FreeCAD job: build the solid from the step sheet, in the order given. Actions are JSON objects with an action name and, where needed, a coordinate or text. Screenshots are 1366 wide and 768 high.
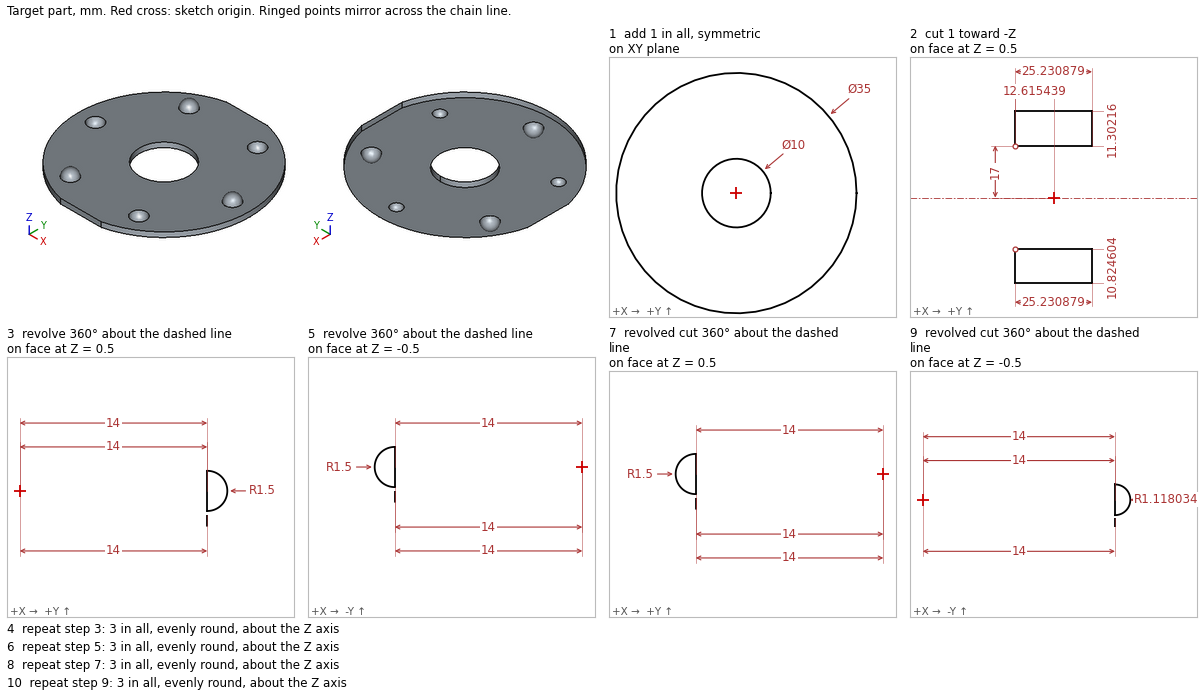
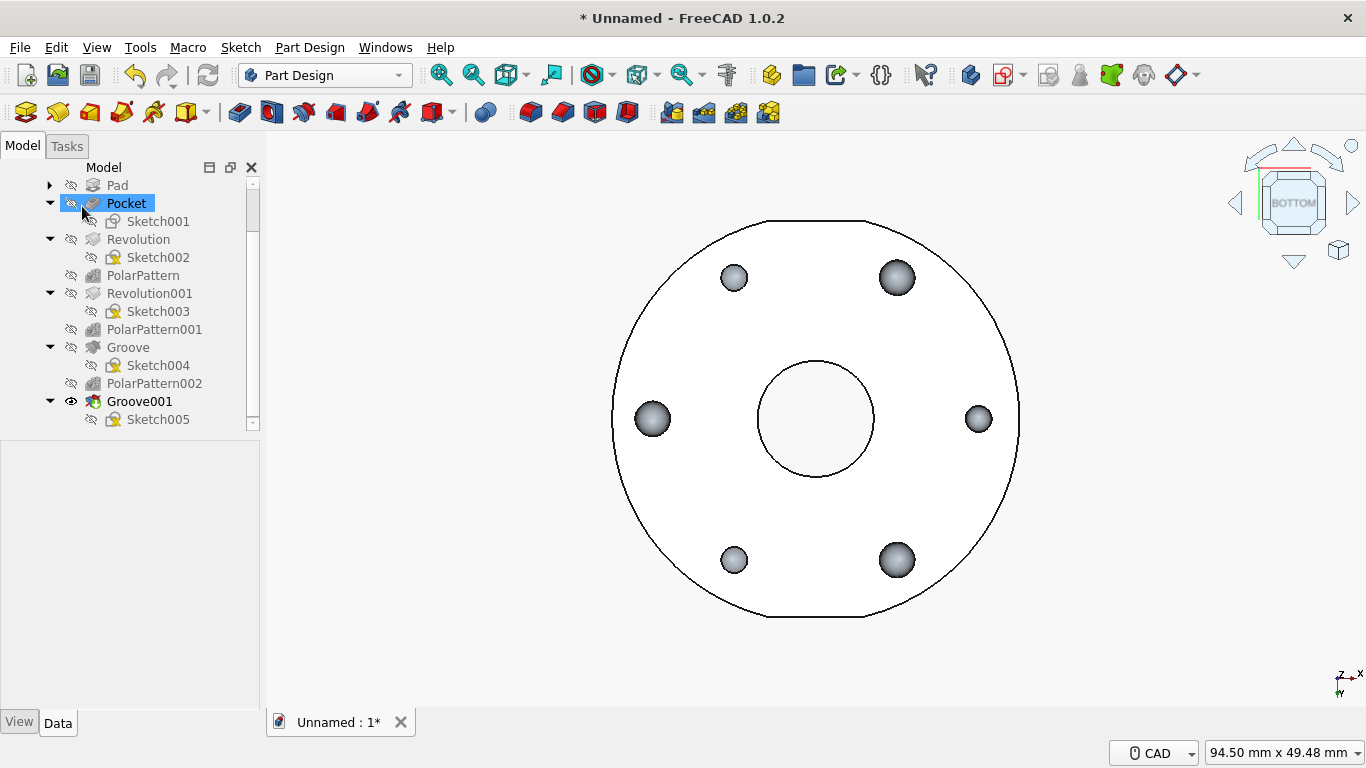
{"action": "left_click", "coordinate": [116, 401]}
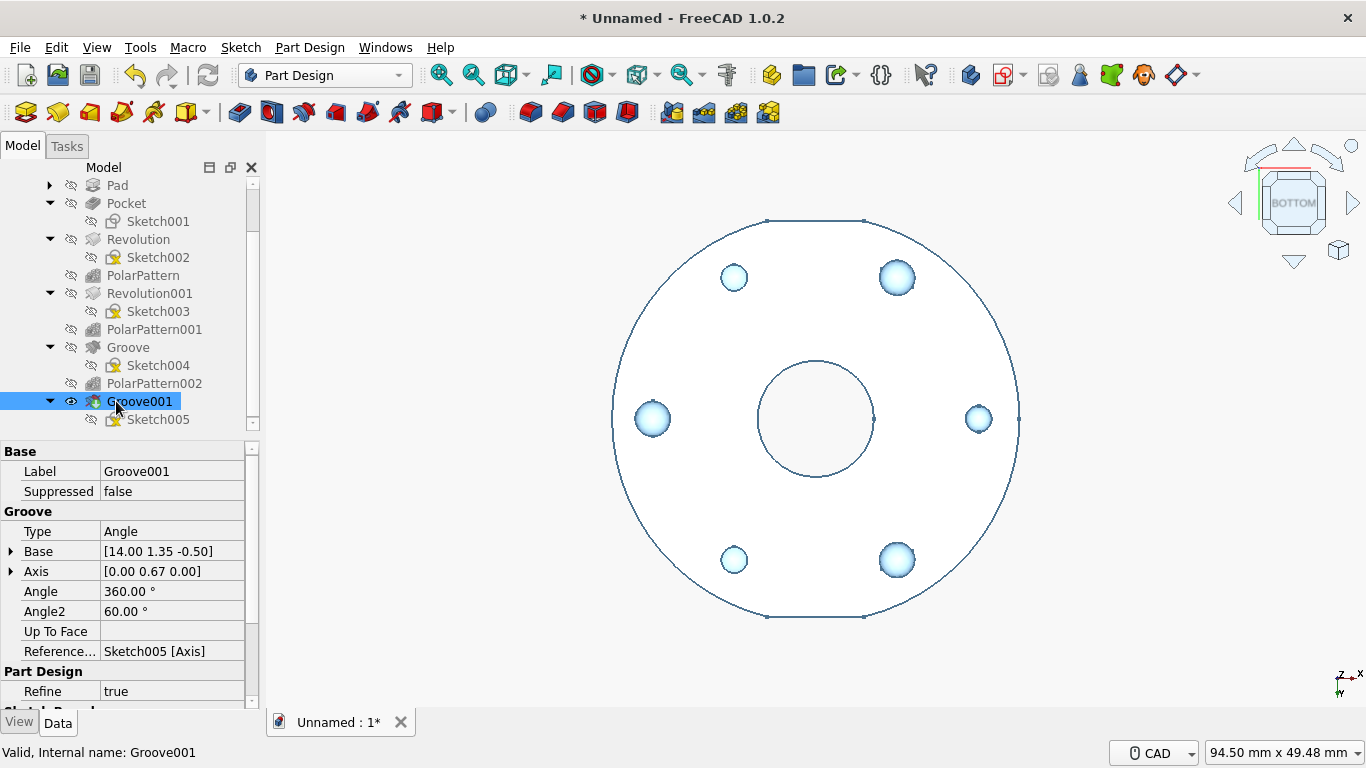
{"action": "left_click", "coordinate": [736, 112]}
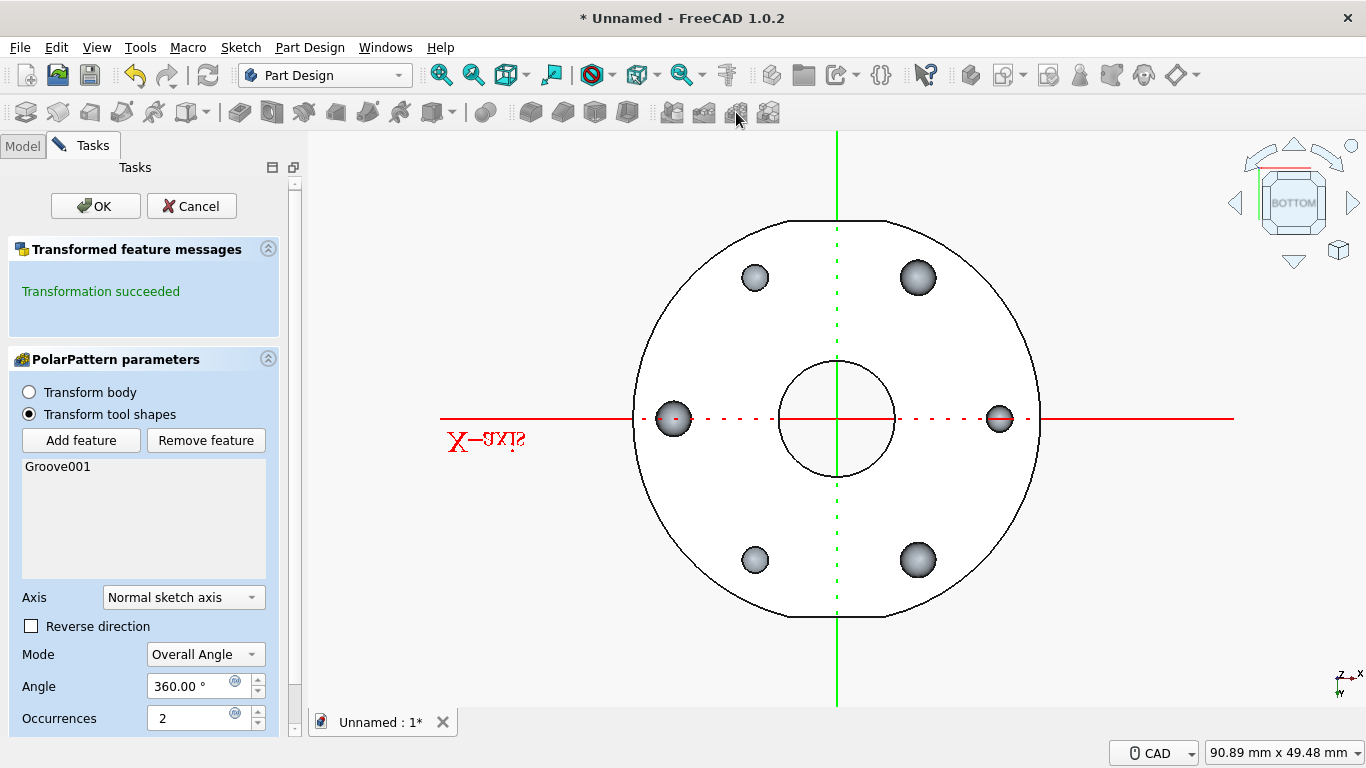
{"action": "left_click", "coordinate": [184, 598]}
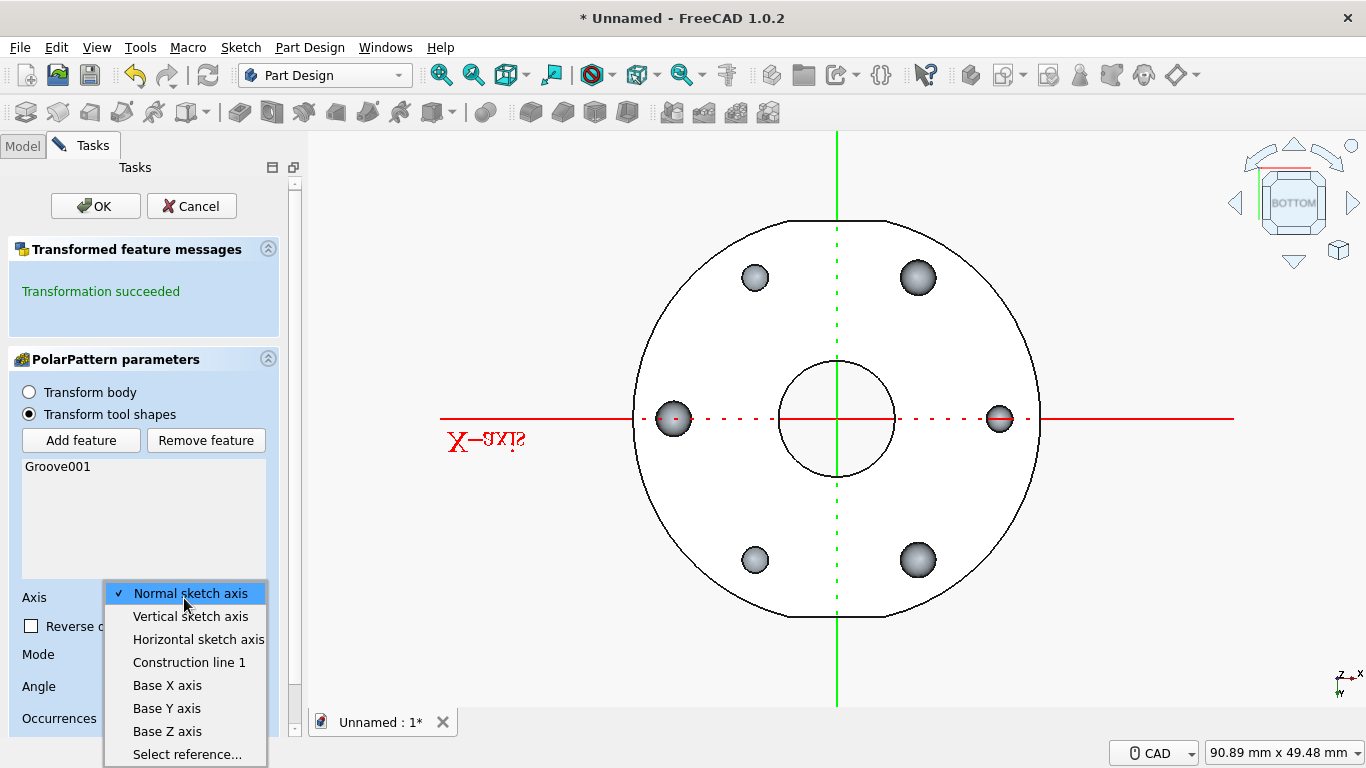
{"action": "left_click", "coordinate": [184, 732]}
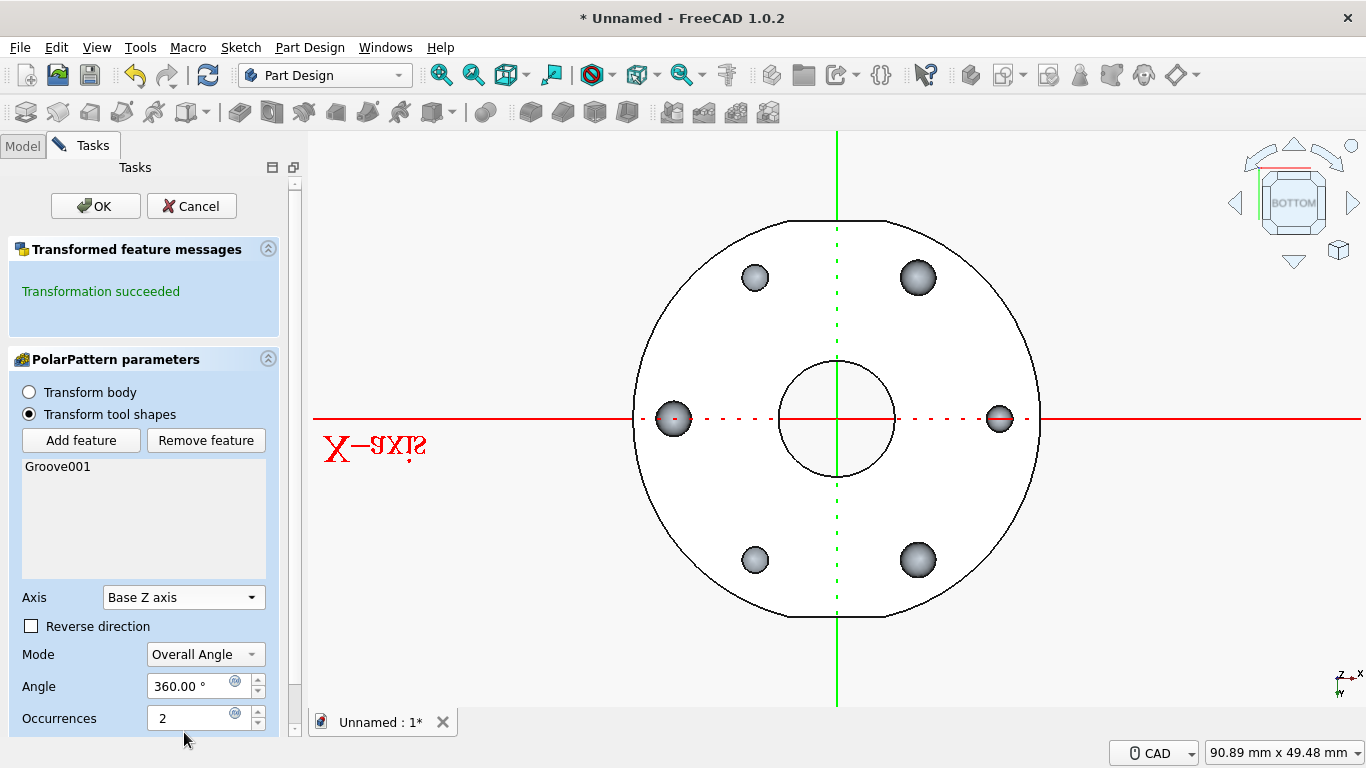
{"action": "triple_click", "coordinate": [198, 718]}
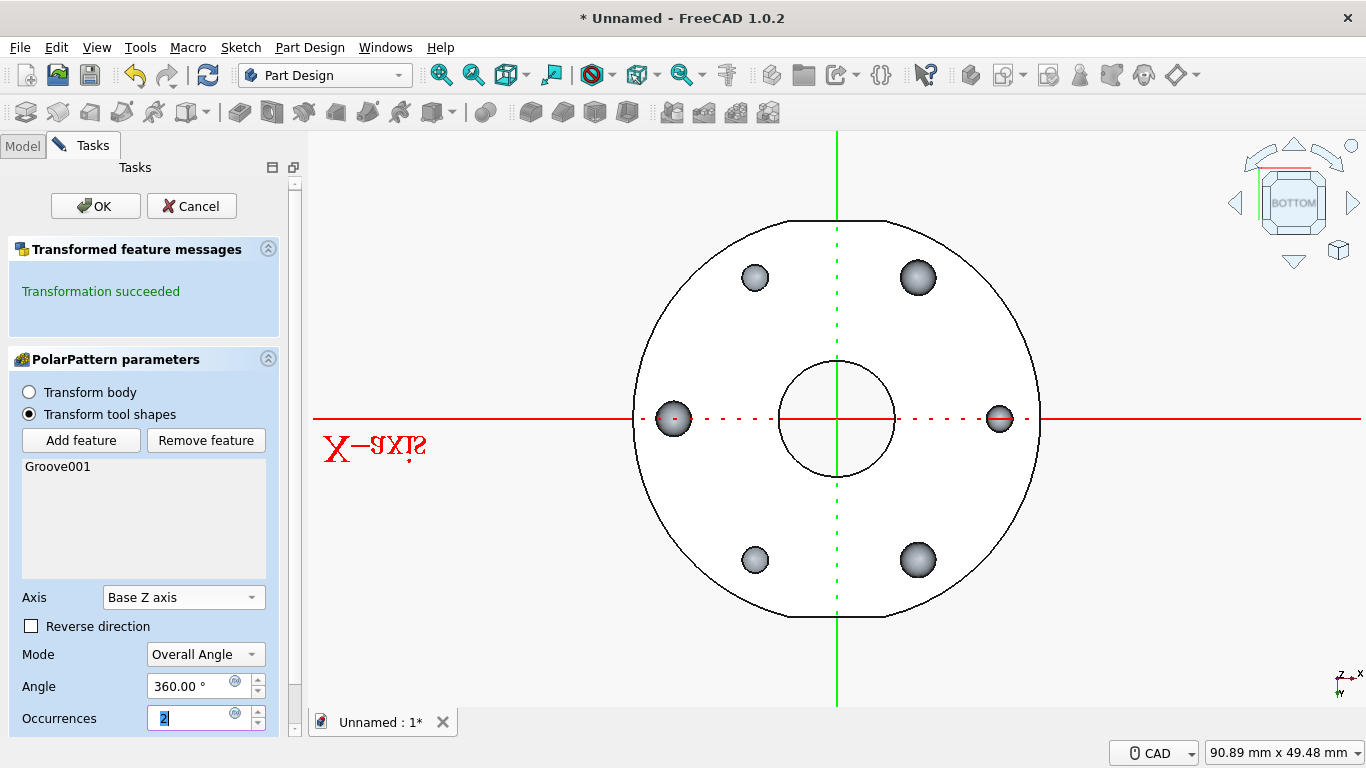
{"action": "type", "text": "3"}
{"action": "key", "text": "Tab"}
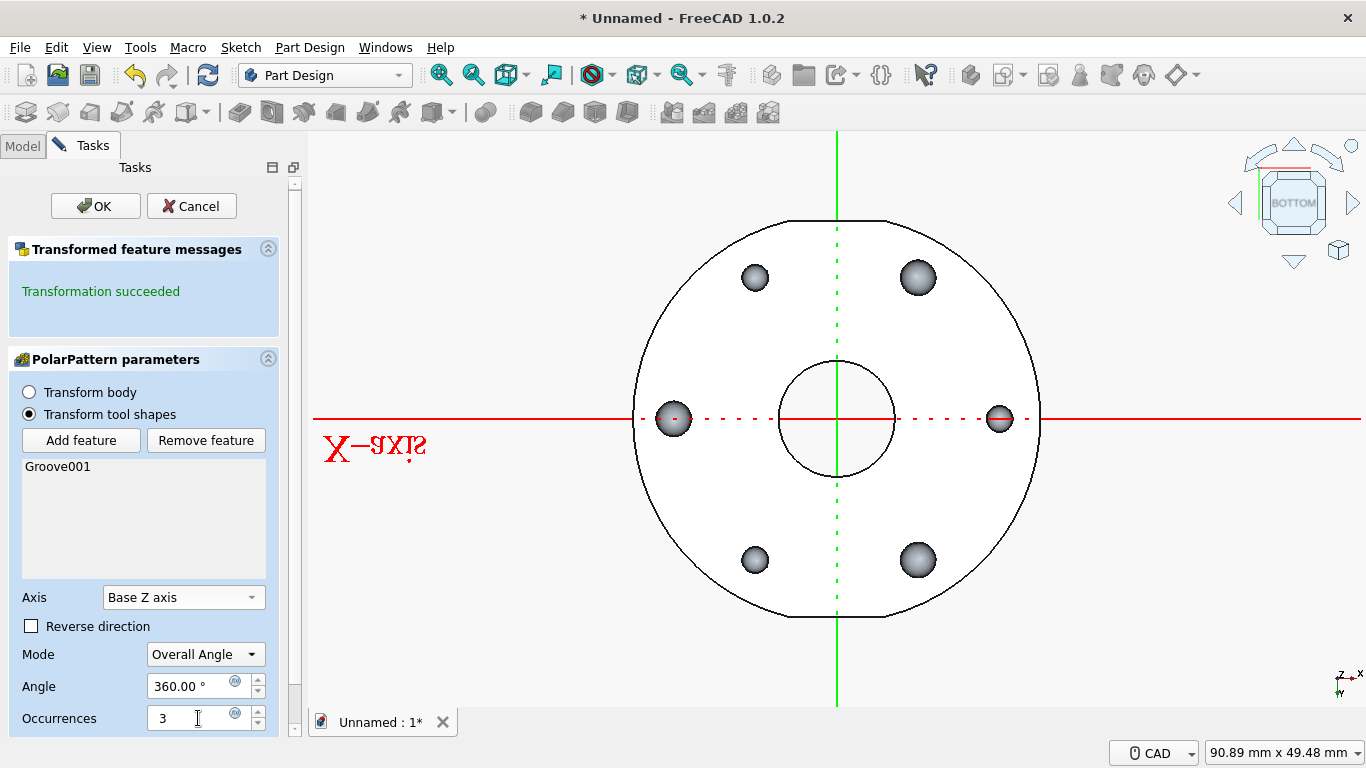
{"action": "left_click", "coordinate": [96, 206]}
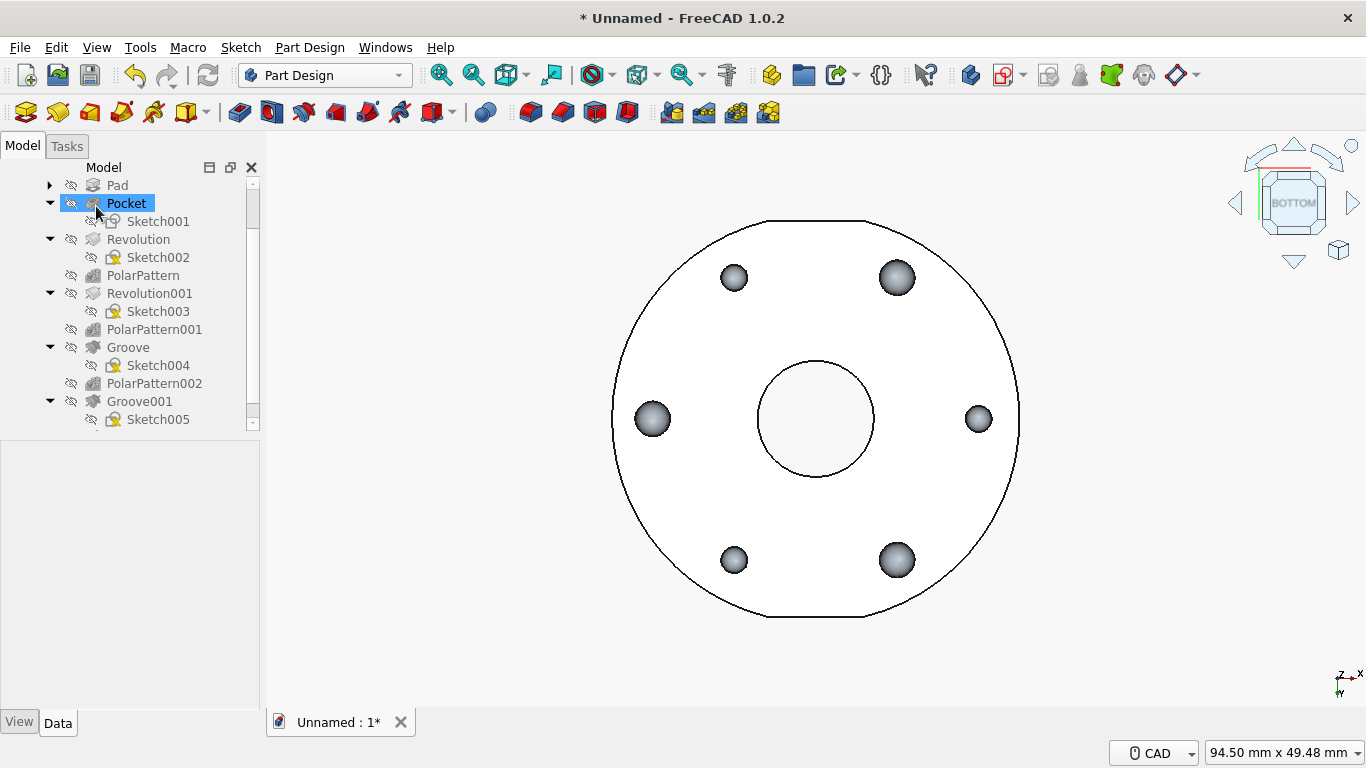
{"action": "key", "text": "0"}